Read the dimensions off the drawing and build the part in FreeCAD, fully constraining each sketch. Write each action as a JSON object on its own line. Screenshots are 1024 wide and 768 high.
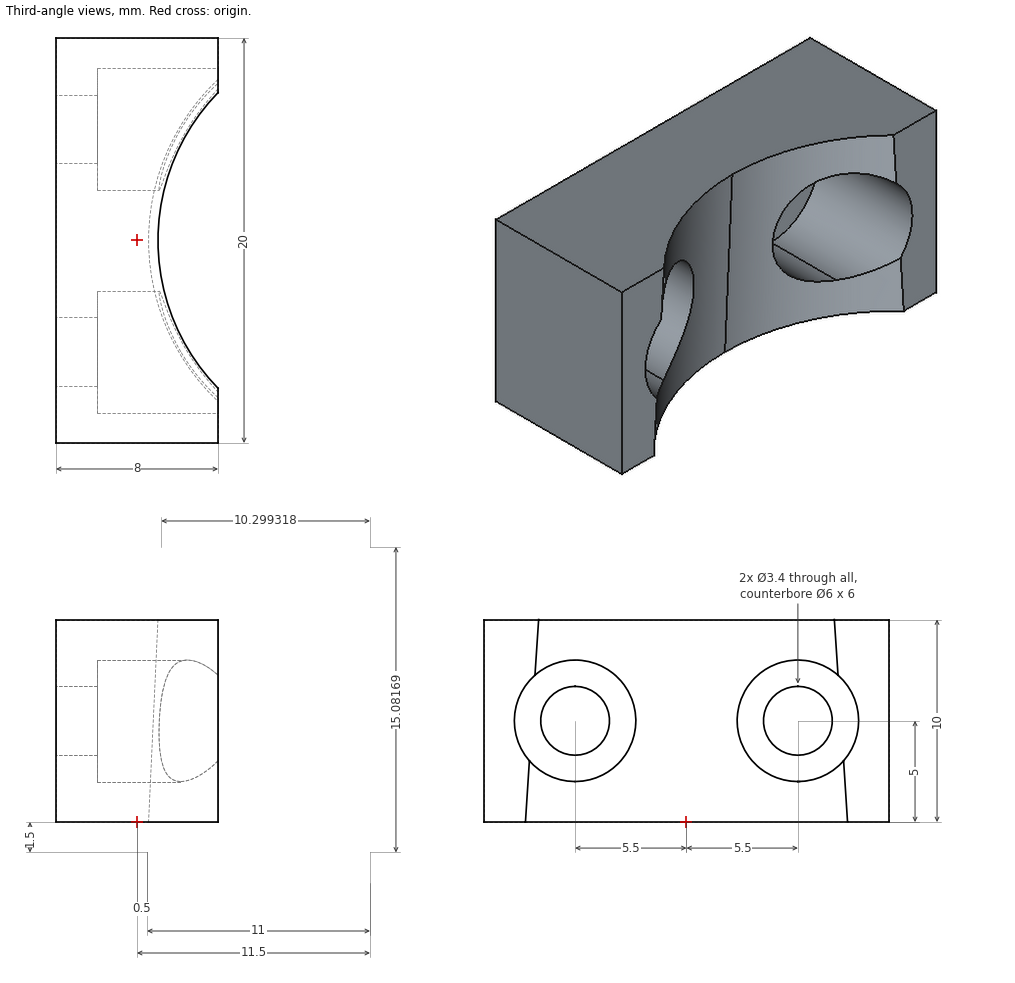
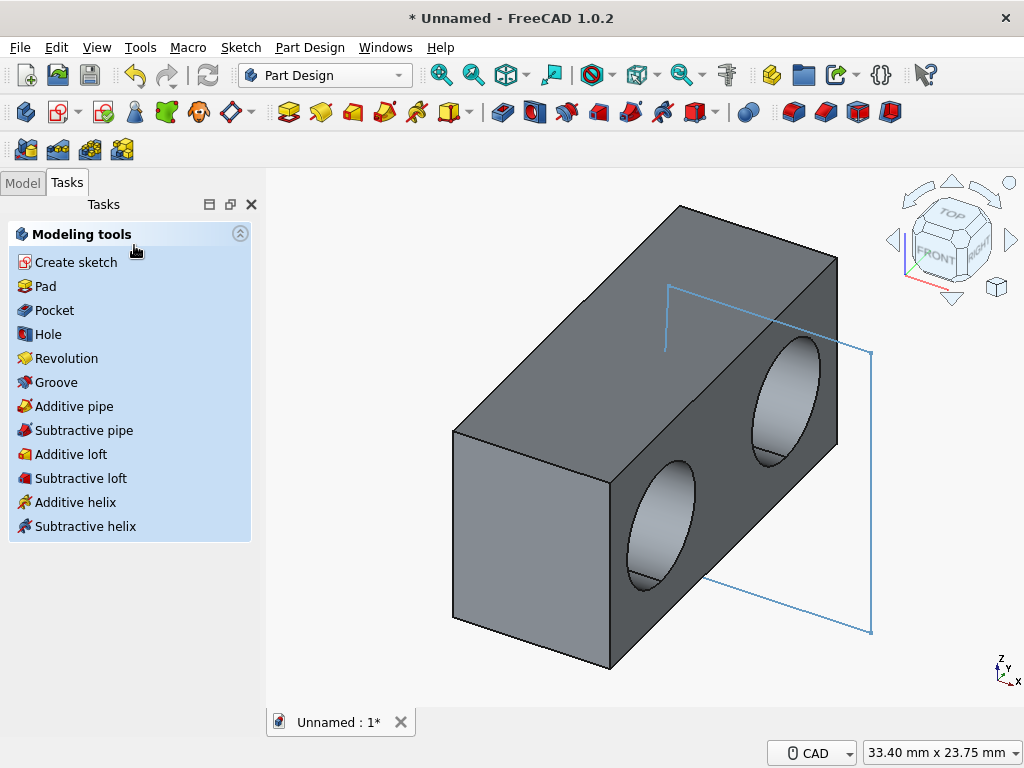
{"action": "left_click", "coordinate": [568, 112]}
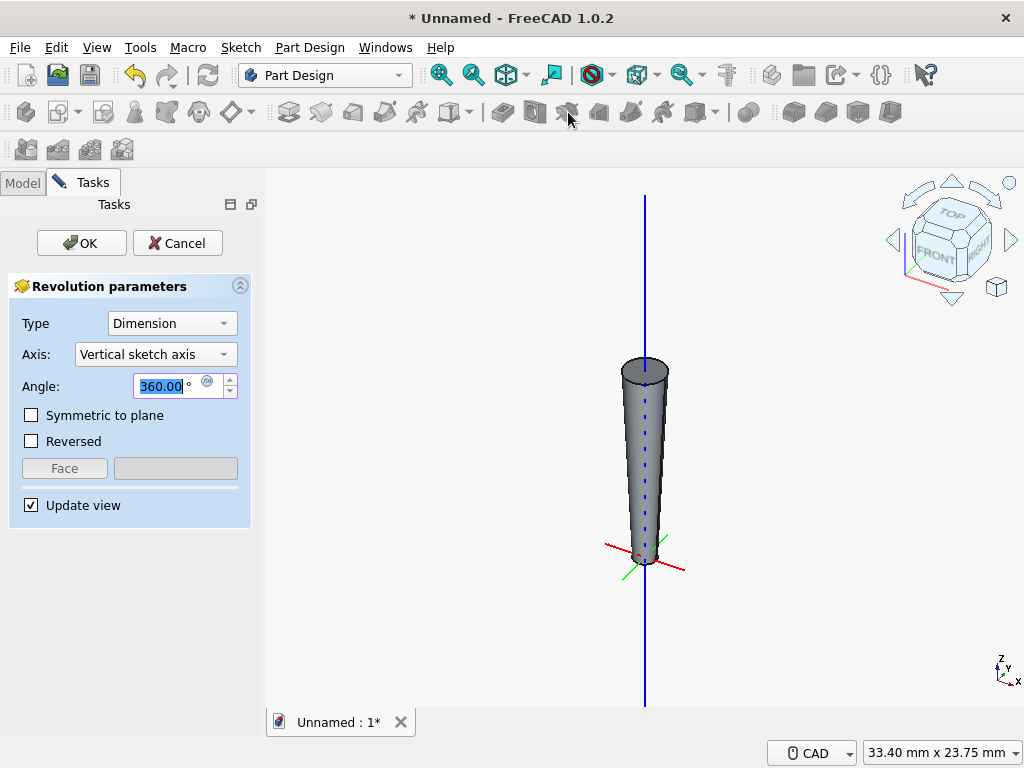
{"action": "left_click", "coordinate": [156, 354]}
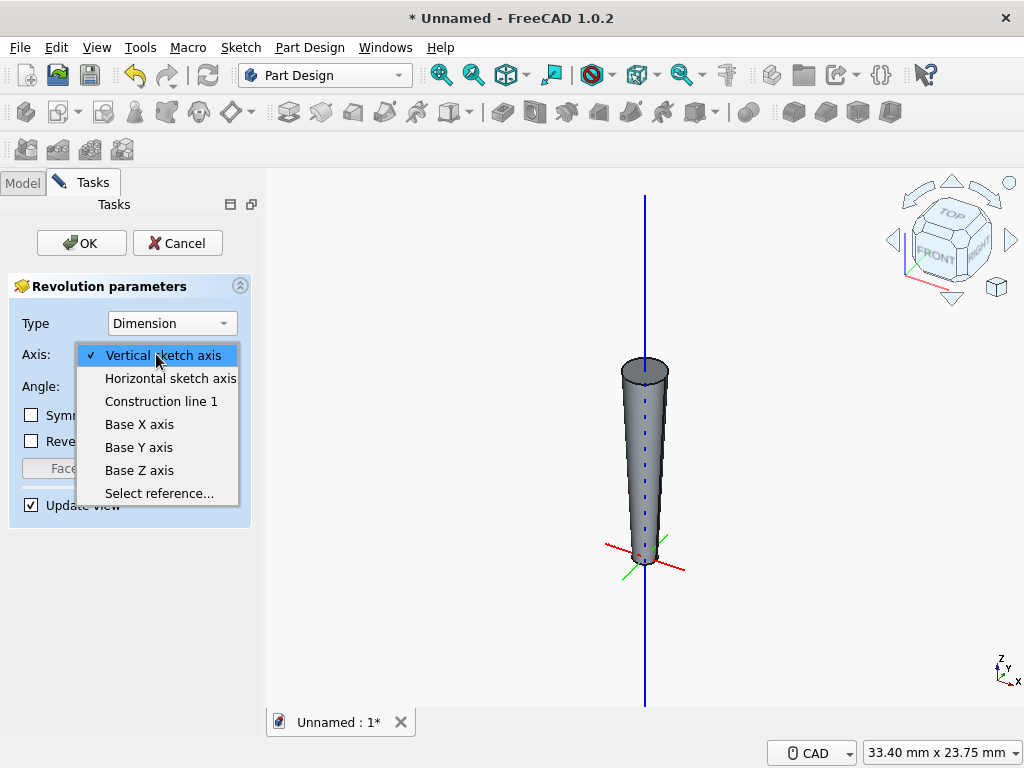
{"action": "left_click", "coordinate": [156, 402]}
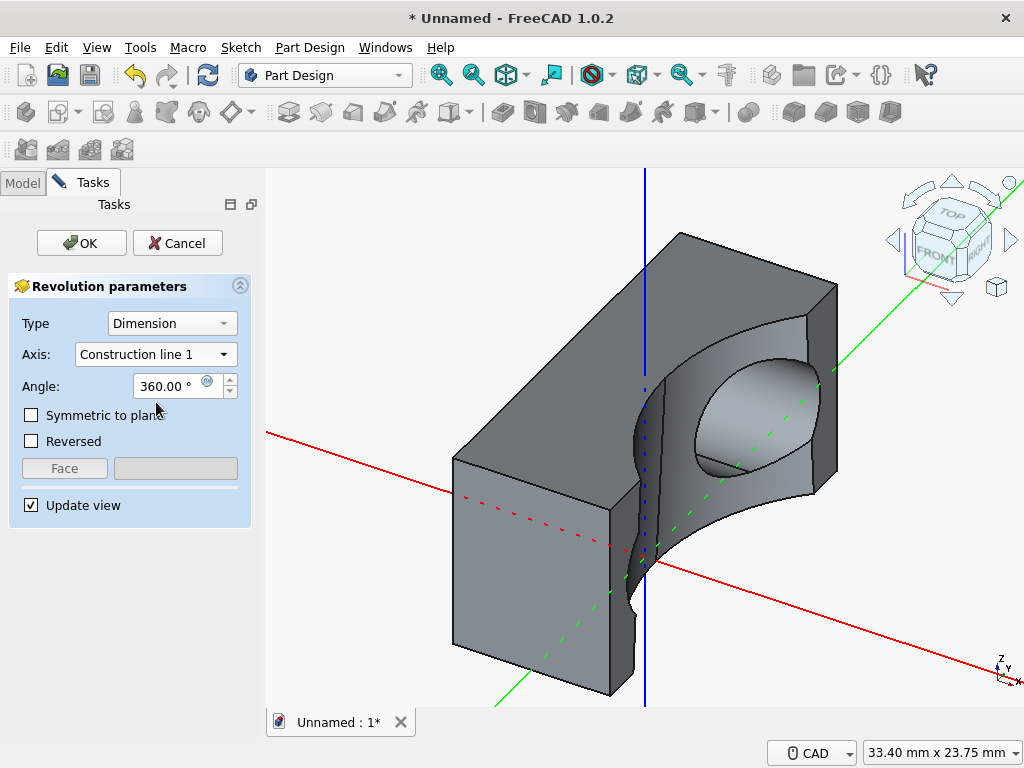
{"action": "left_click", "coordinate": [82, 243]}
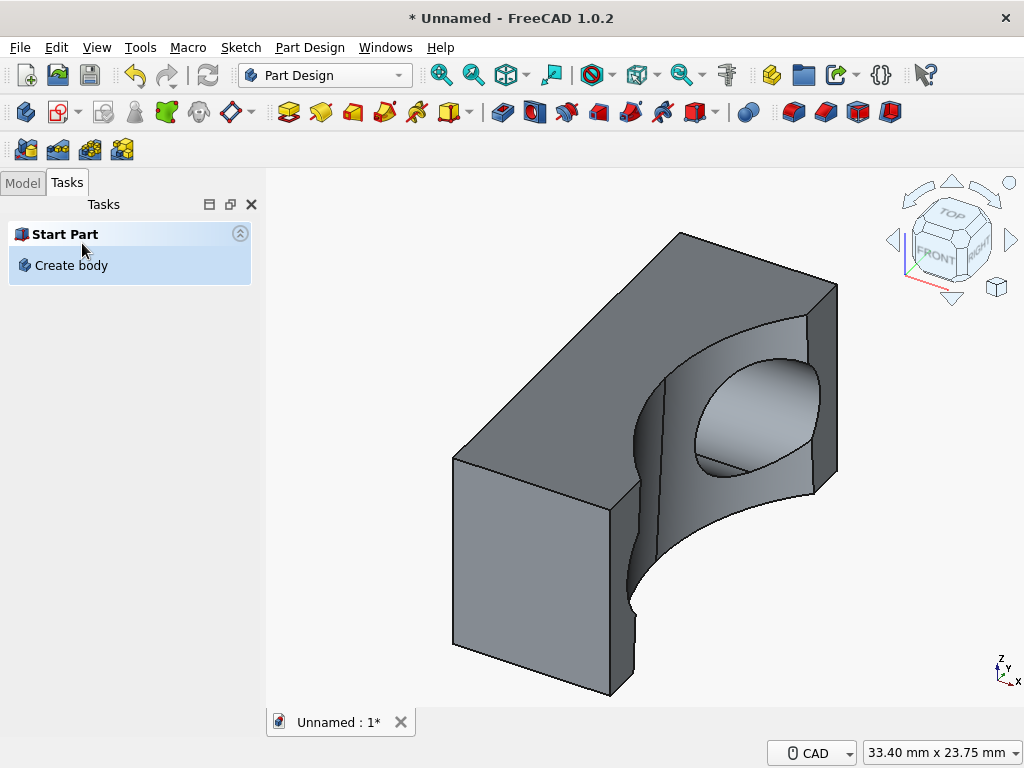
{"action": "key", "text": "0"}